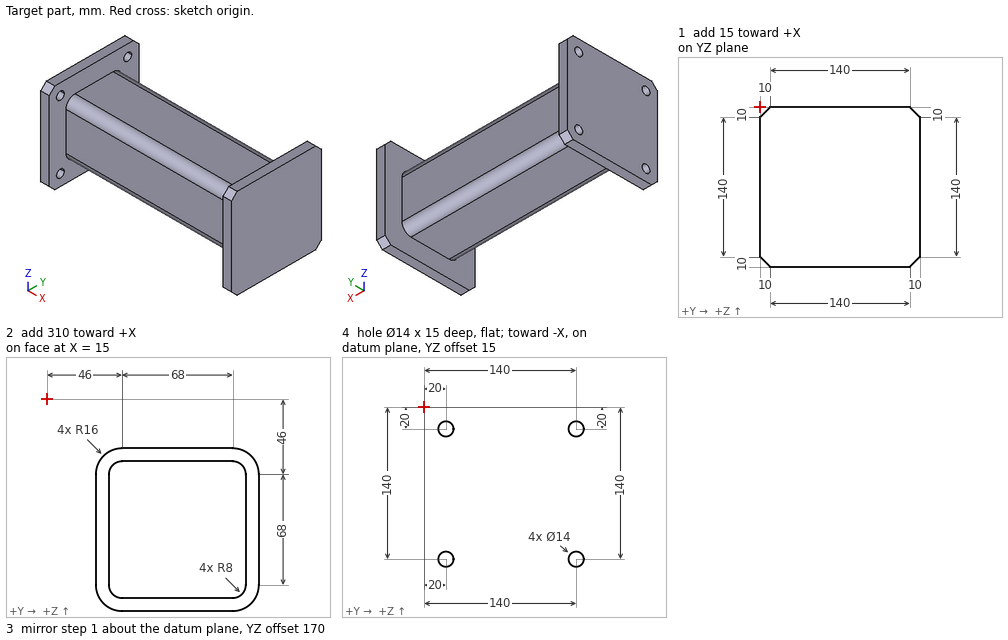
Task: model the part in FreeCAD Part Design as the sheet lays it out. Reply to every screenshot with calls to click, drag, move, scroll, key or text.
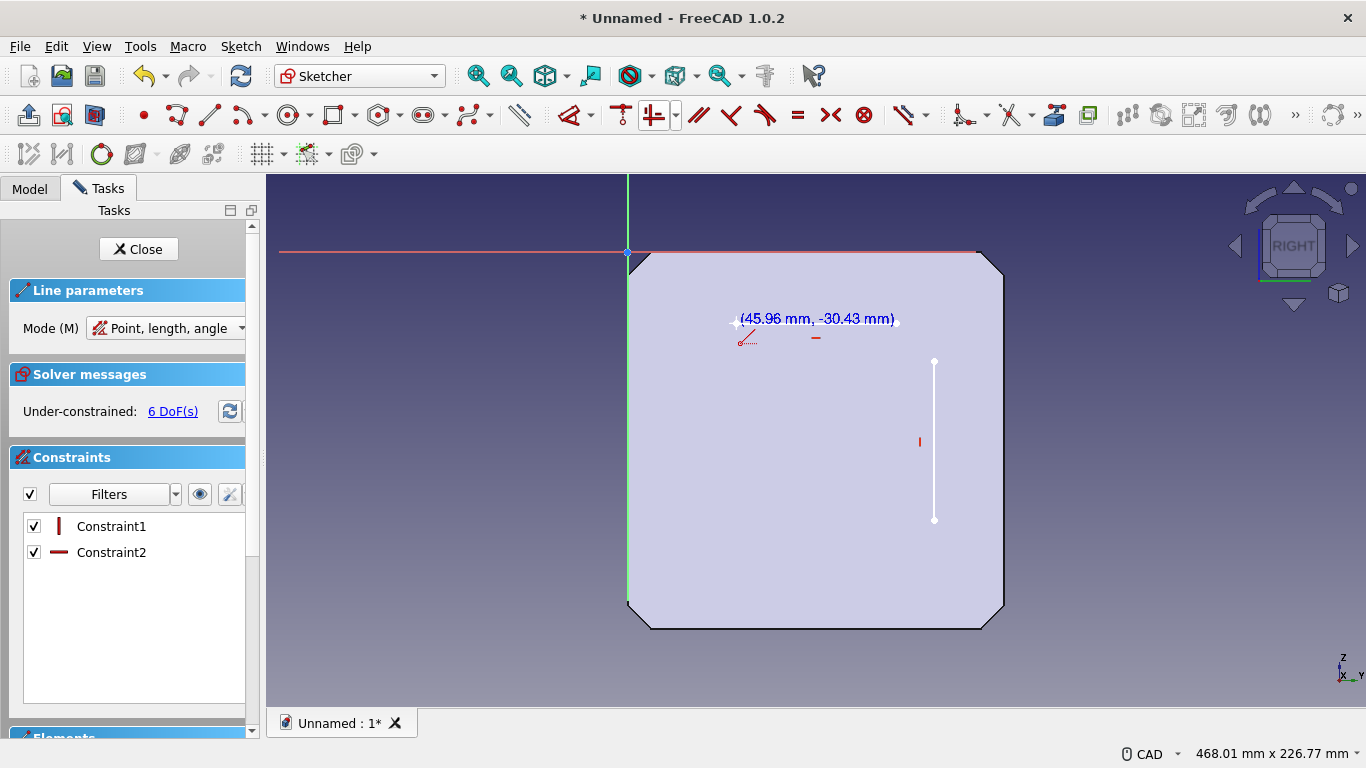
click(698, 361)
click(698, 520)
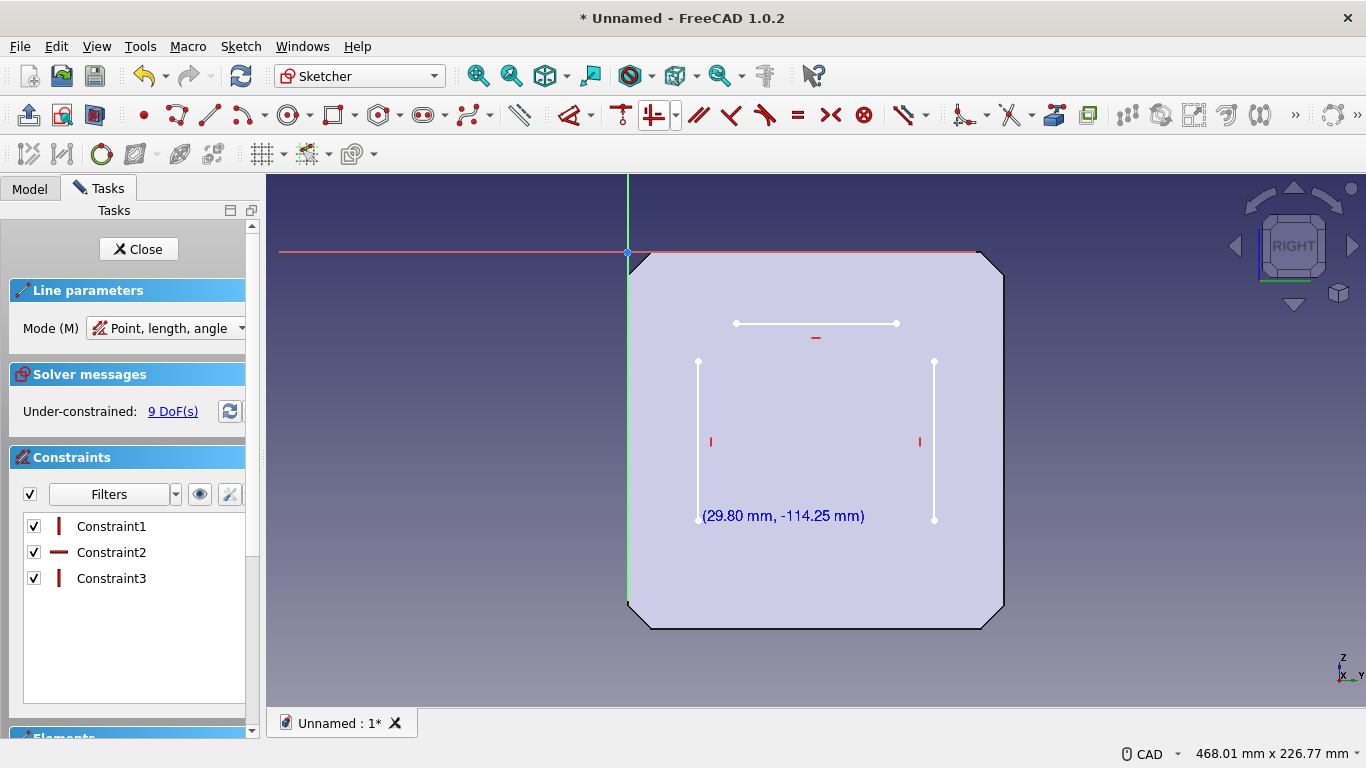
click(736, 558)
click(896, 558)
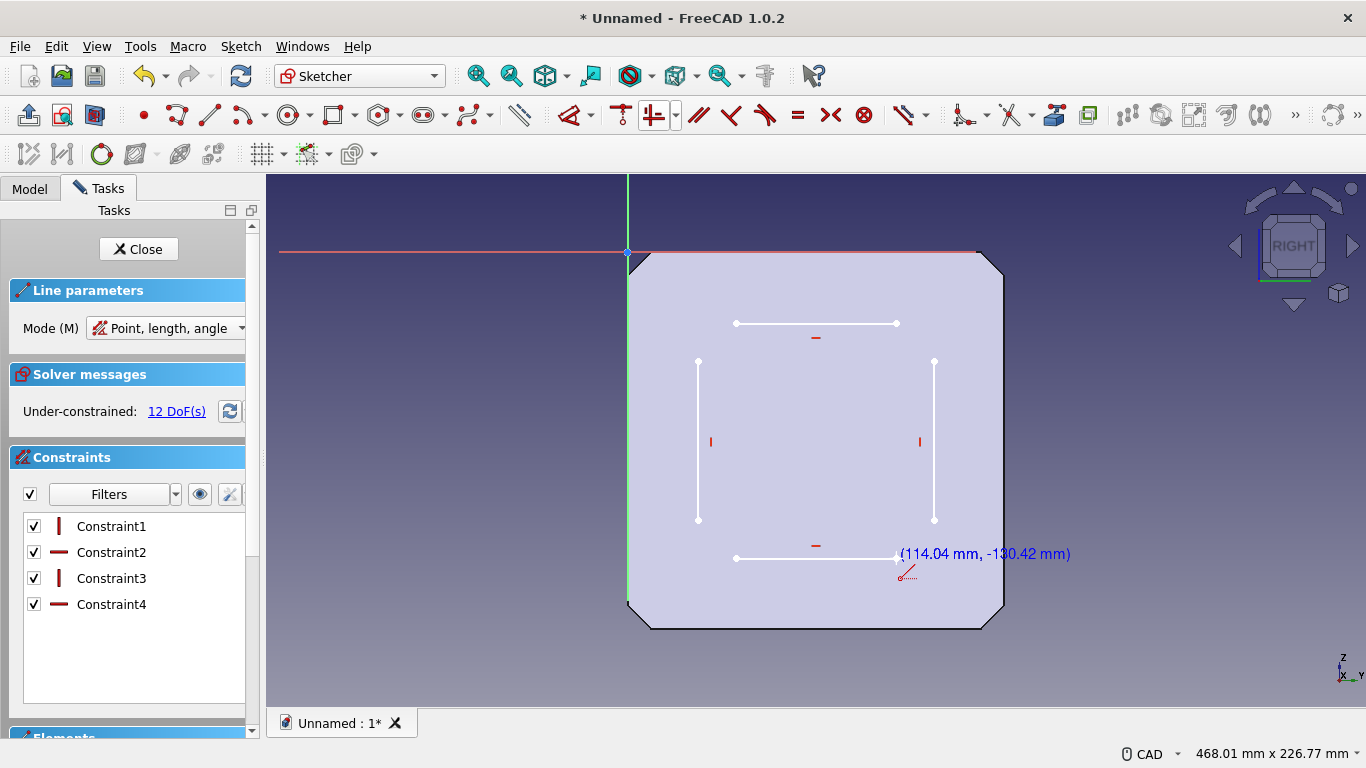
key(g)
key(3)
key(a)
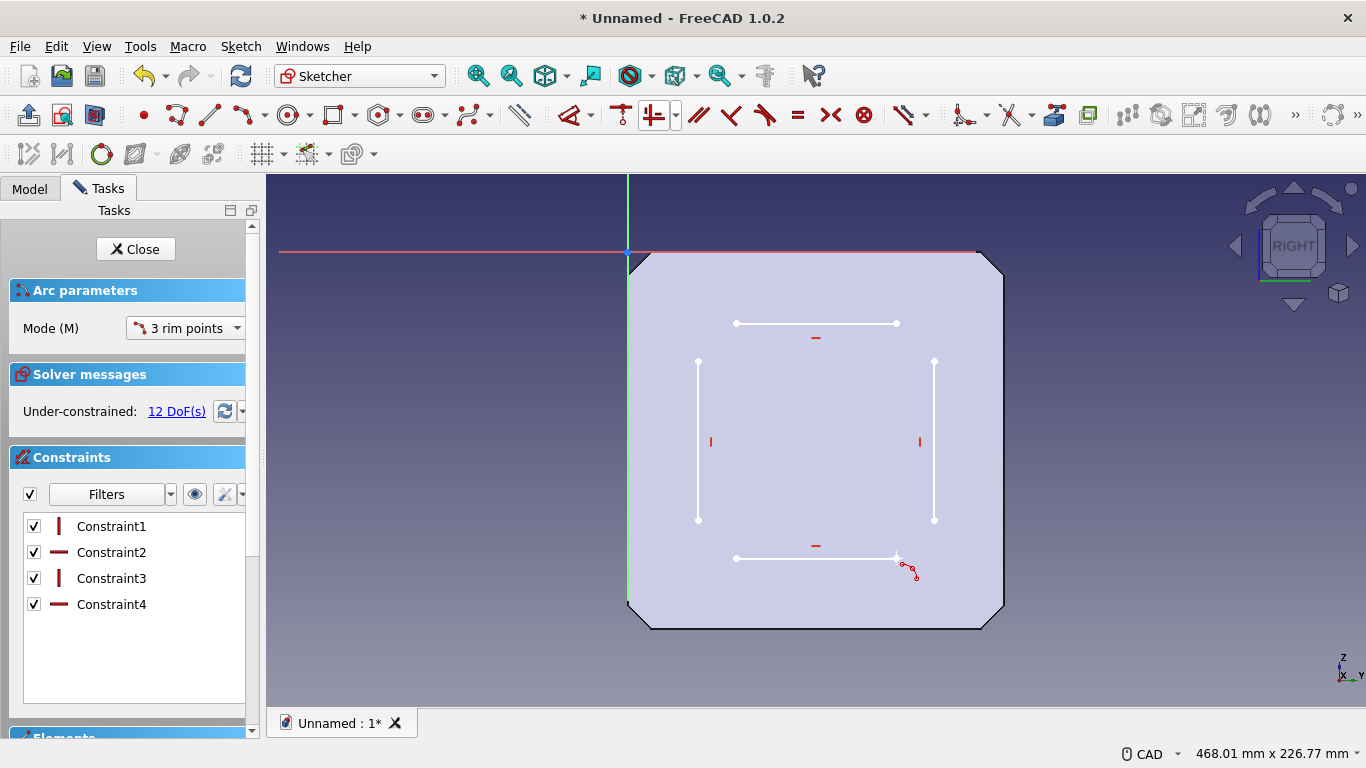
click(934, 362)
click(896, 324)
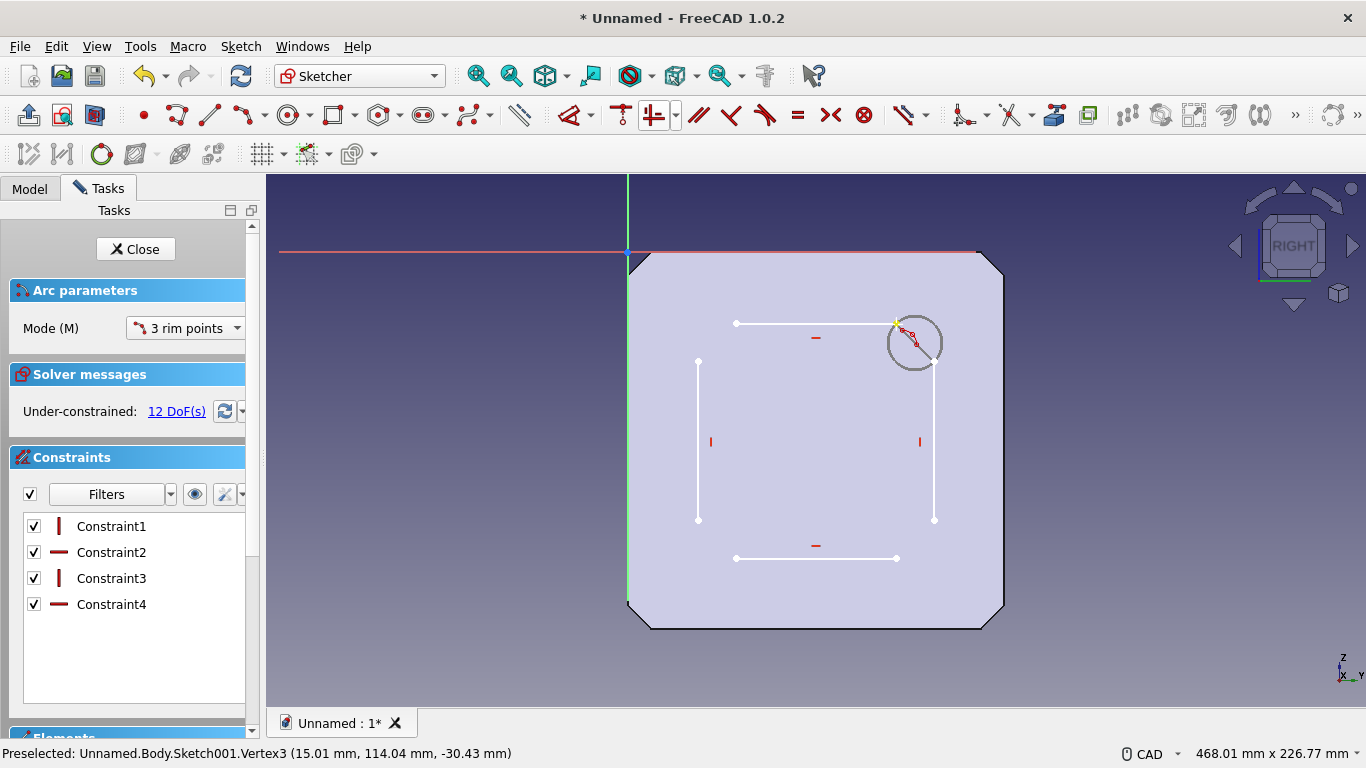
scroll(923, 334, up, 2)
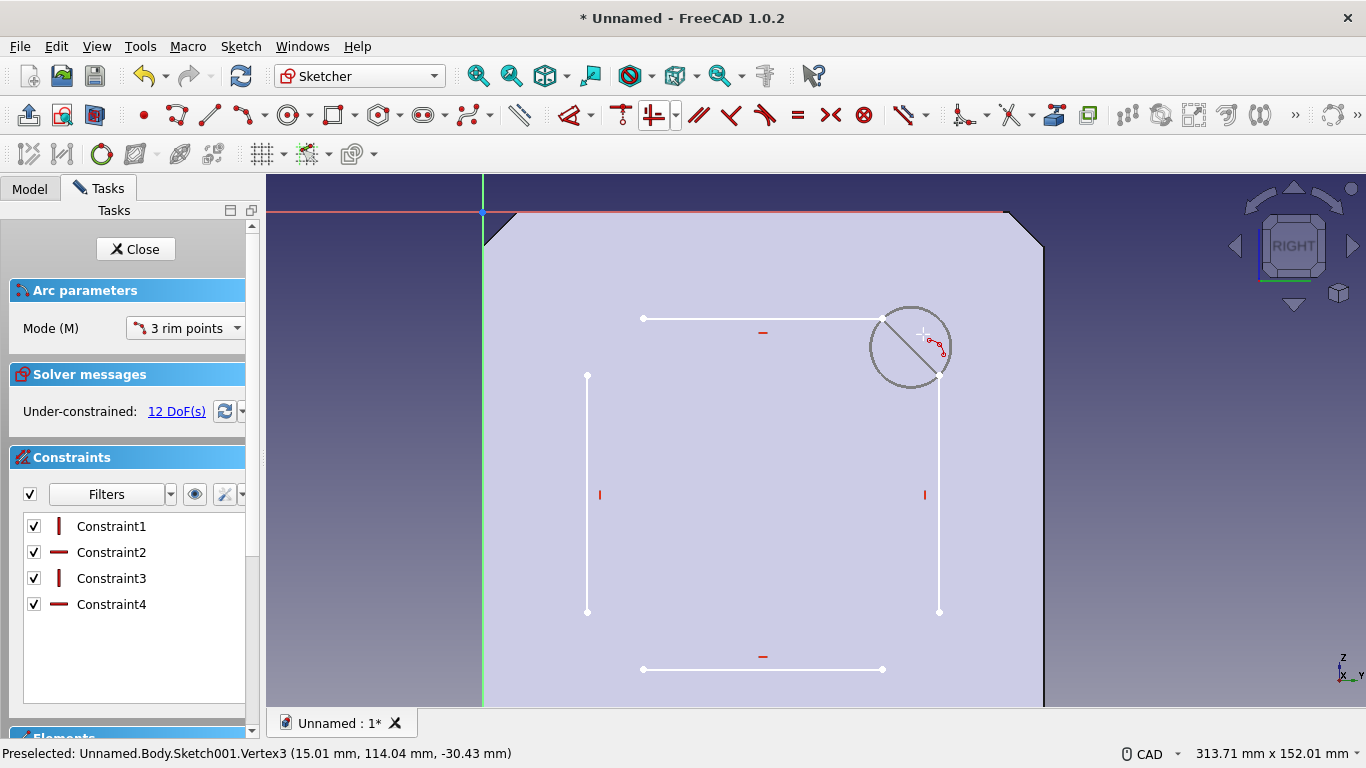
click(922, 334)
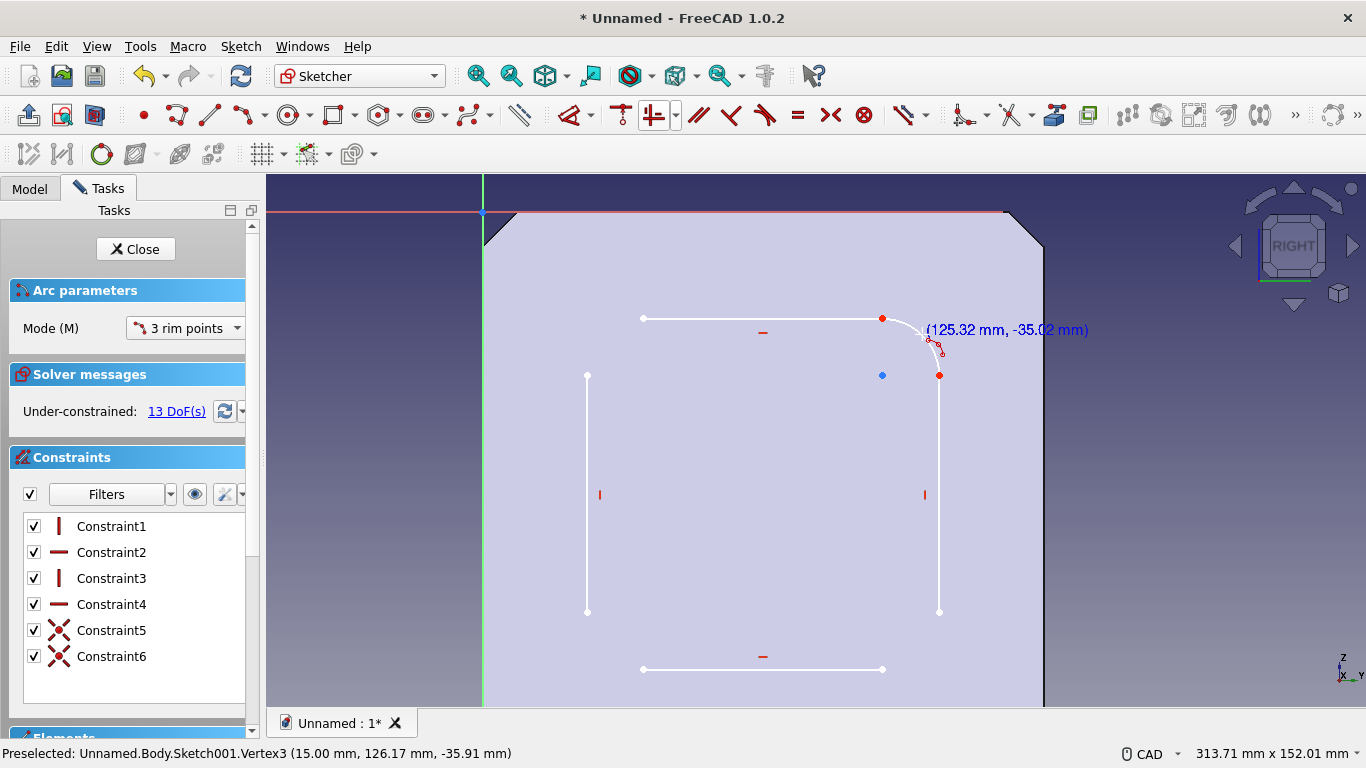
click(644, 319)
click(587, 376)
click(604, 334)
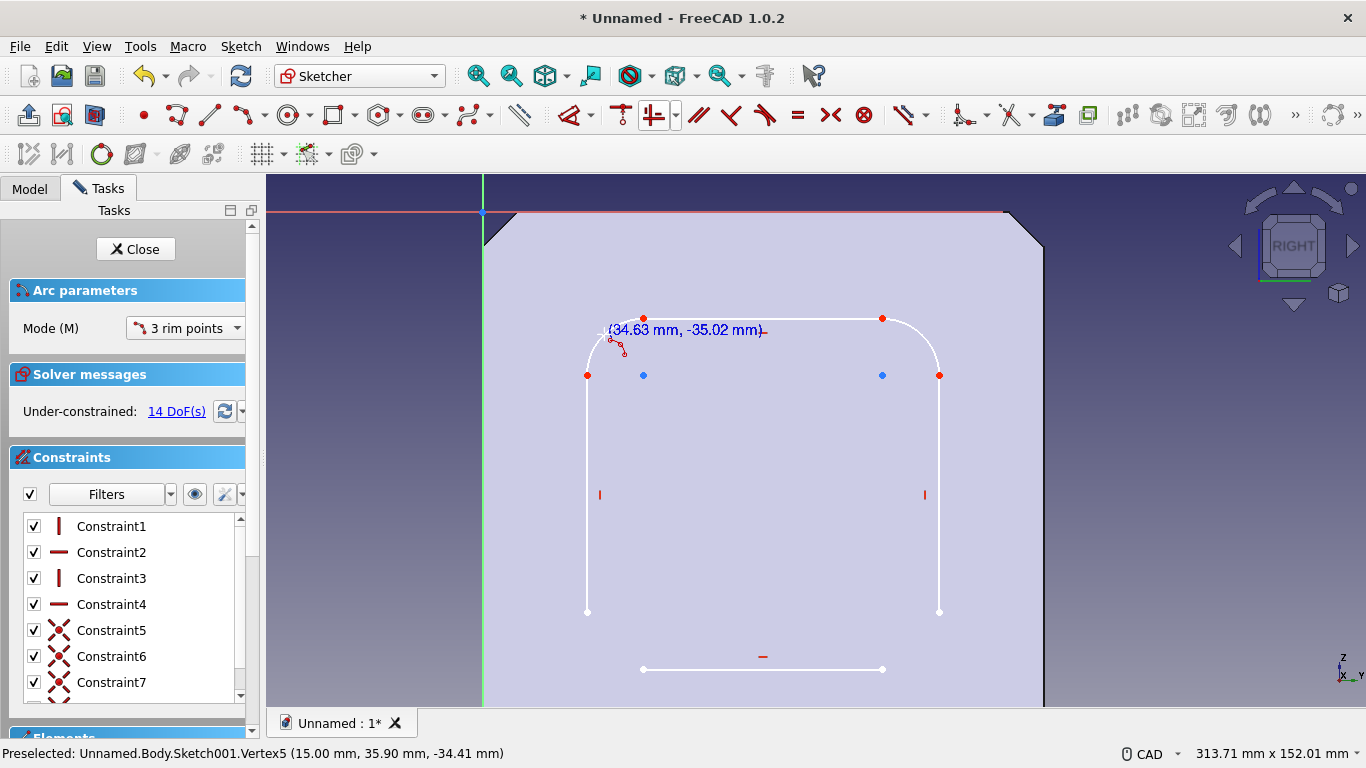
click(587, 613)
click(644, 670)
click(604, 652)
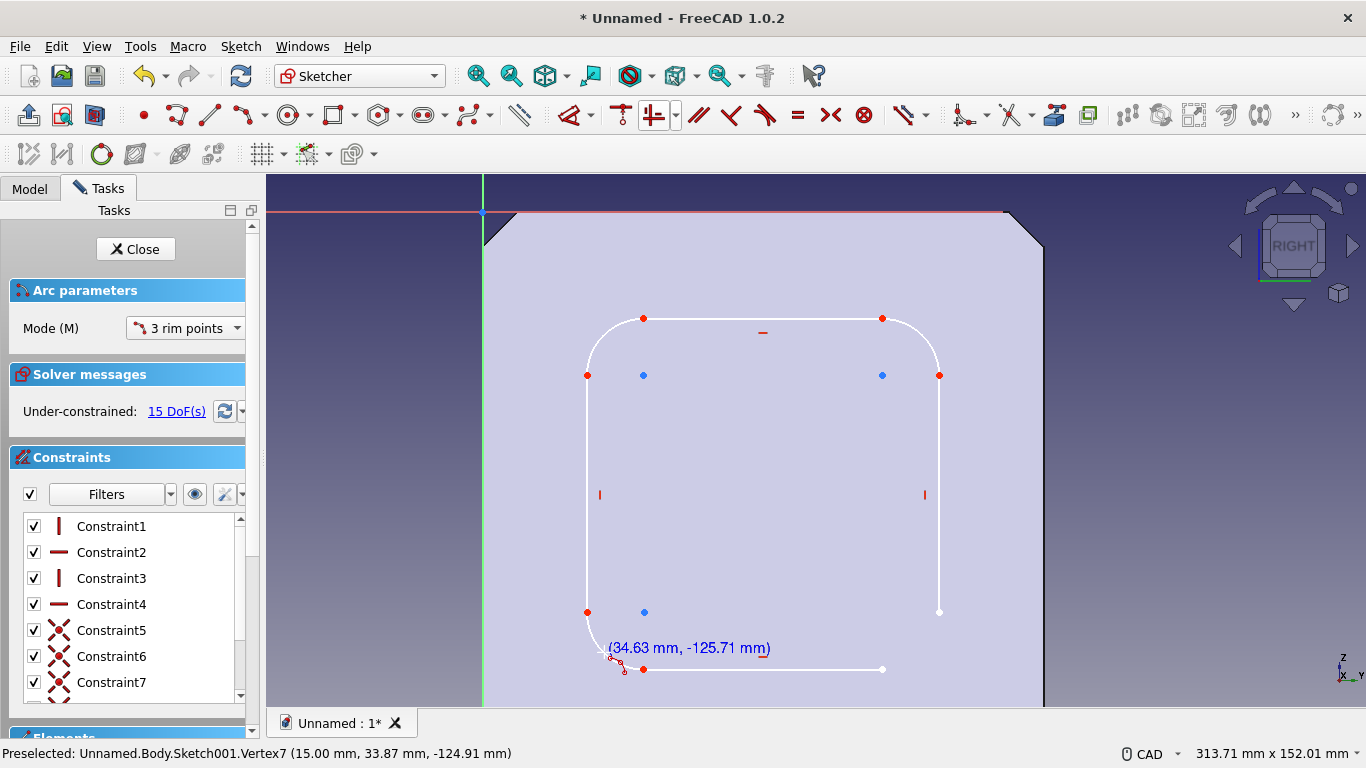
click(882, 670)
click(939, 613)
click(922, 652)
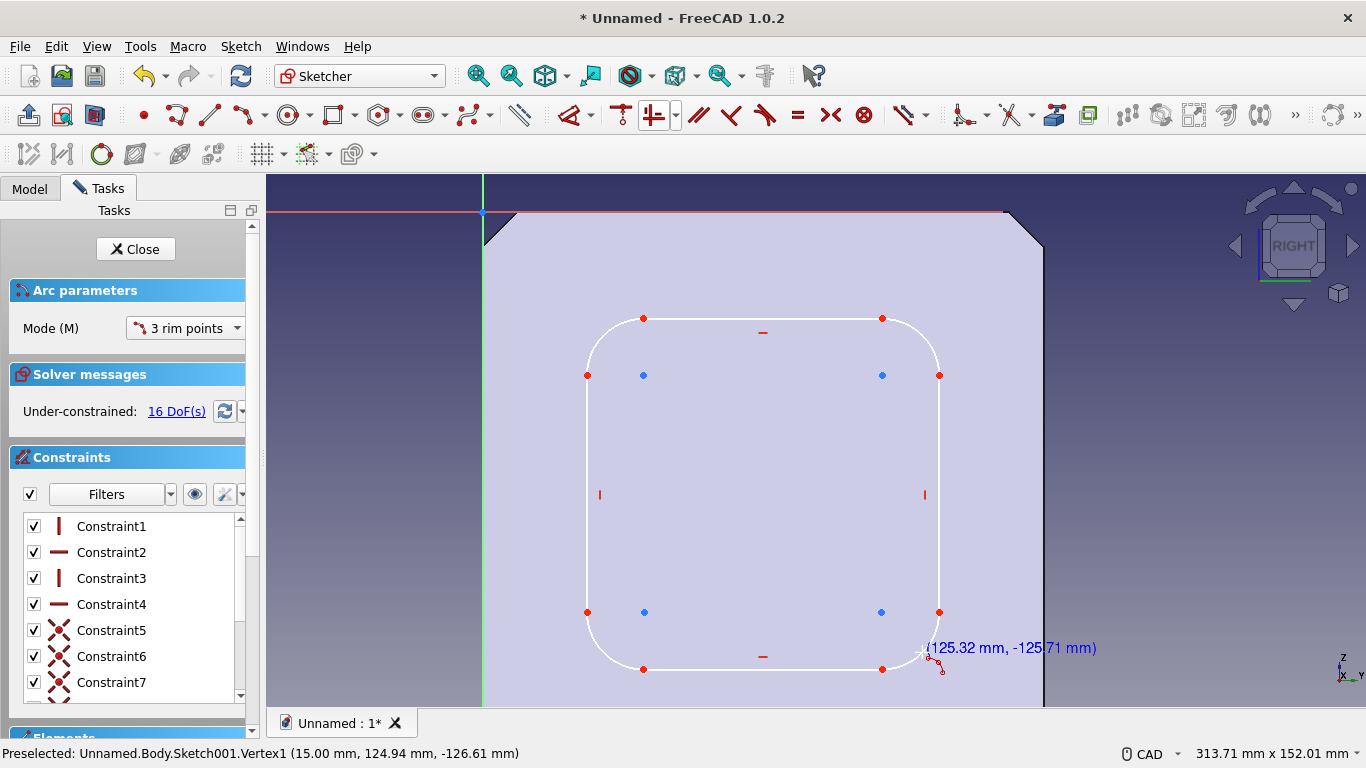
click(210, 116)